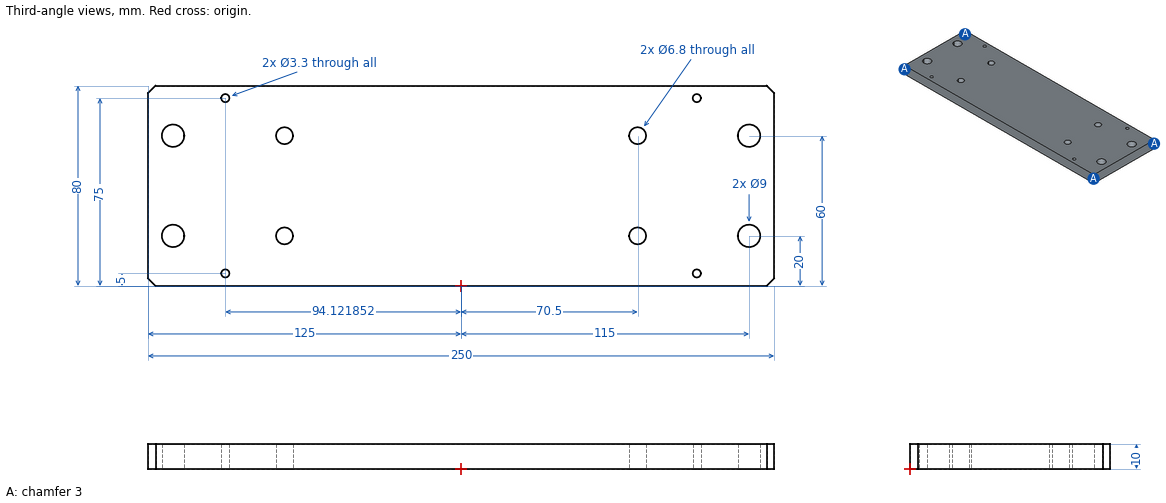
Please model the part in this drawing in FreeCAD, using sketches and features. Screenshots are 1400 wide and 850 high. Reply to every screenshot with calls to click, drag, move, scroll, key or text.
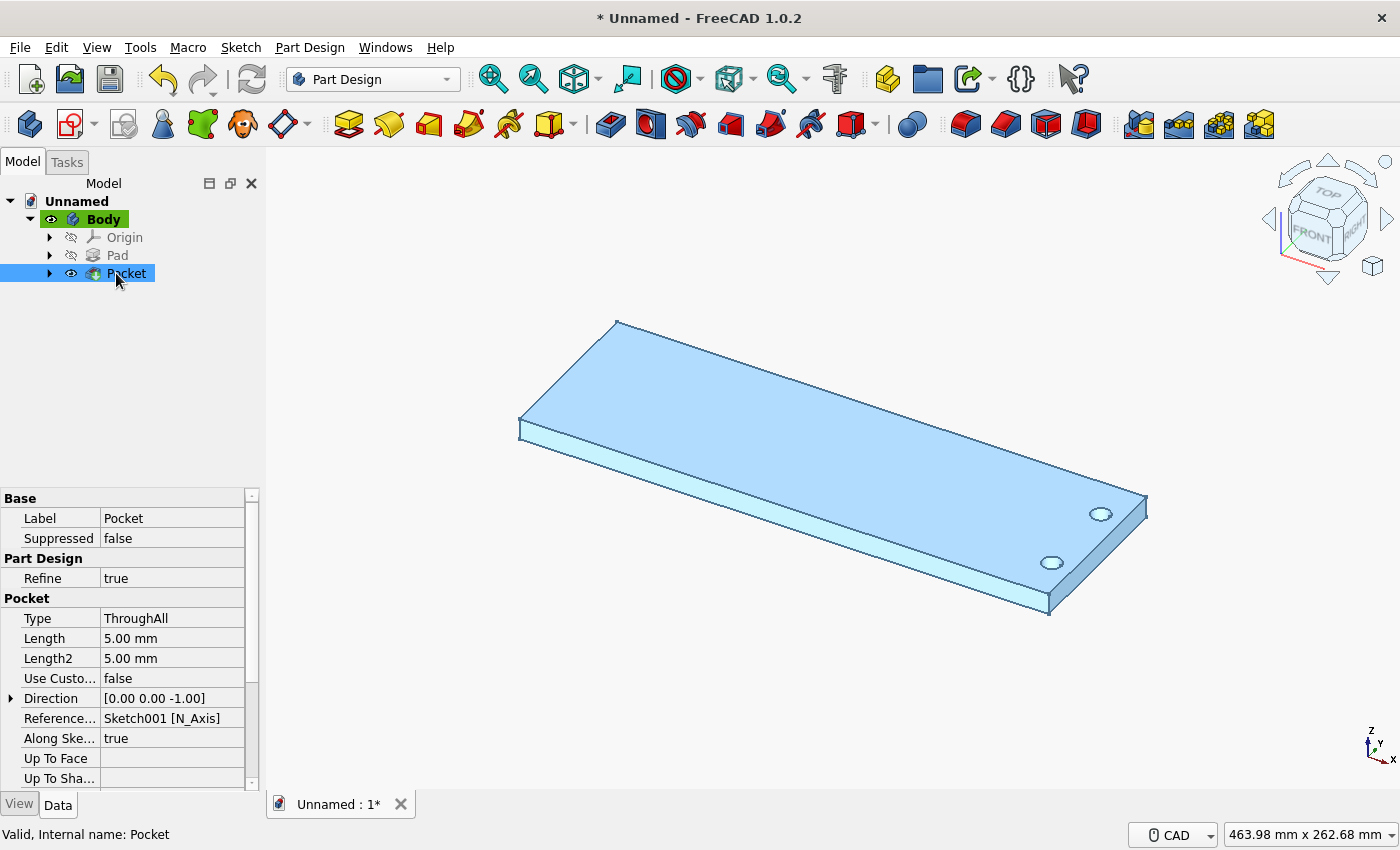
click(1140, 124)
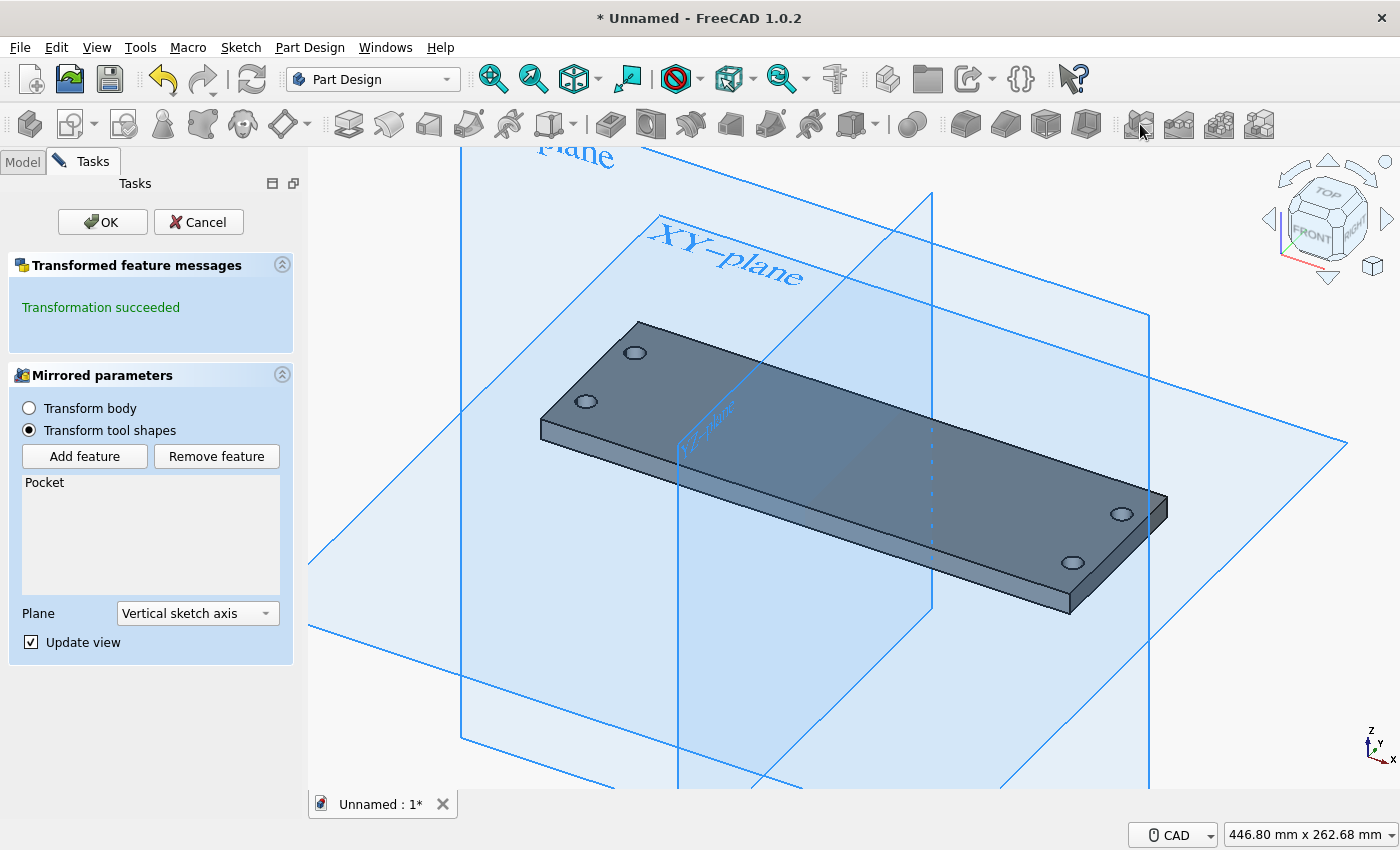
click(198, 614)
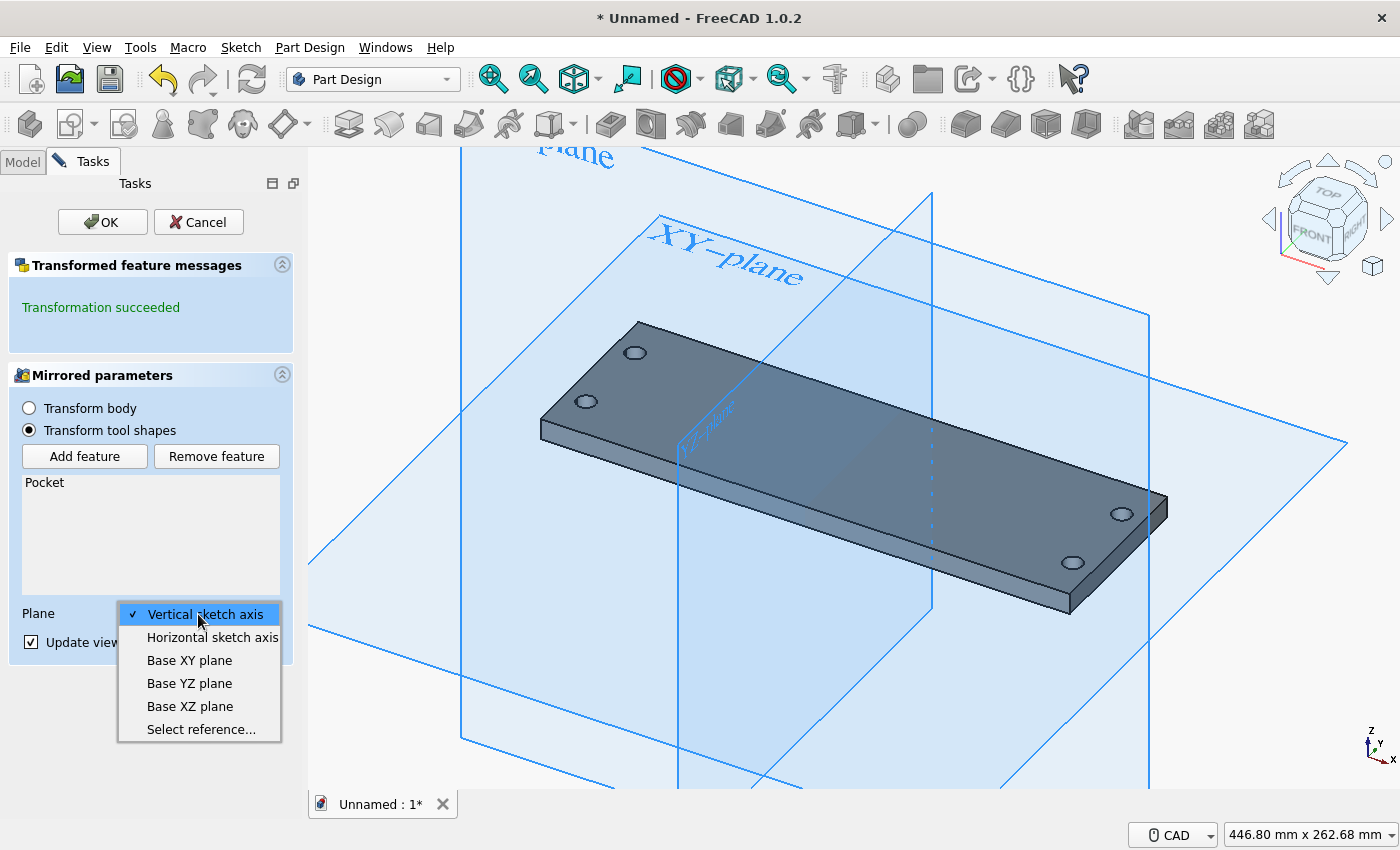
click(198, 684)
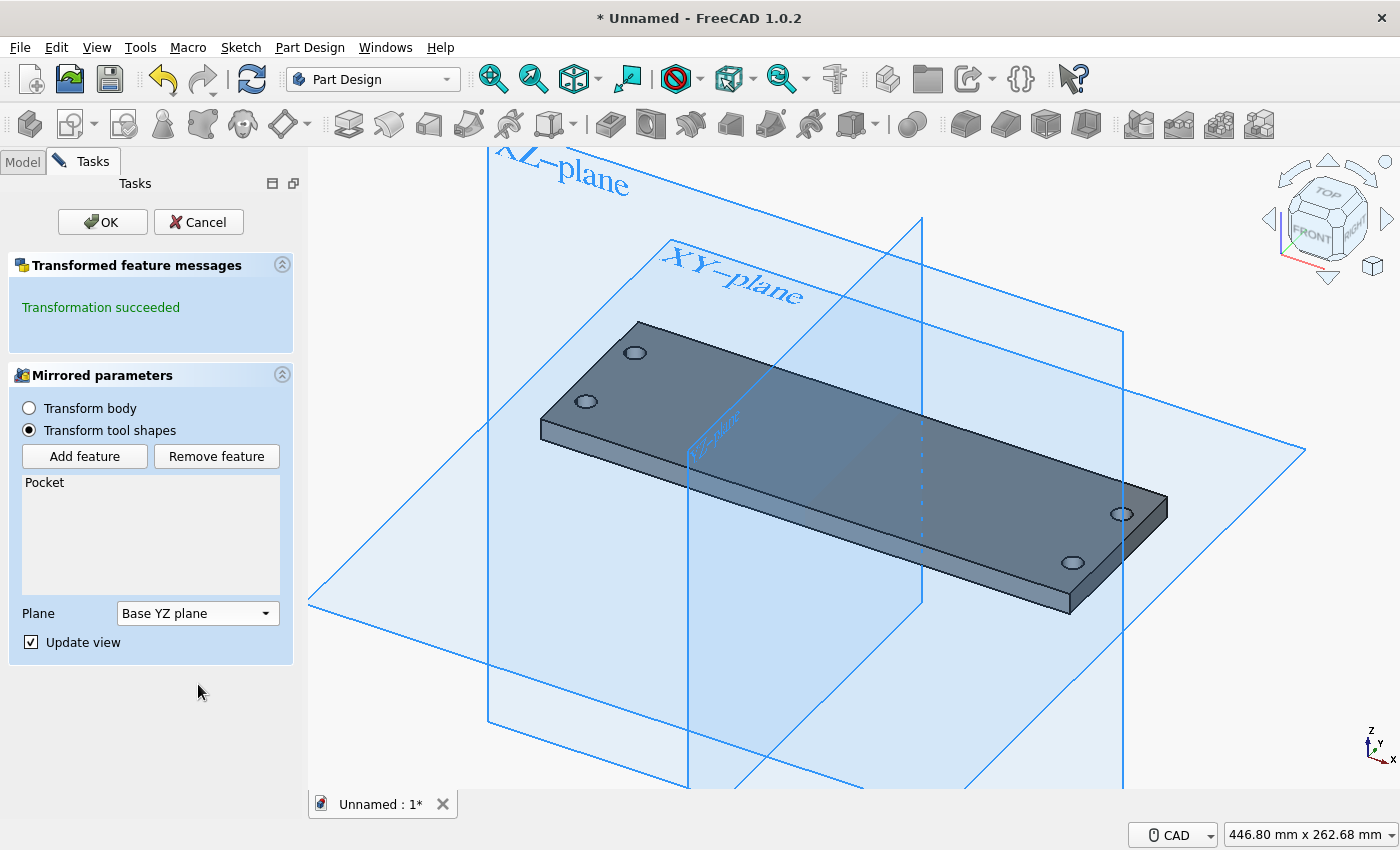
click(103, 222)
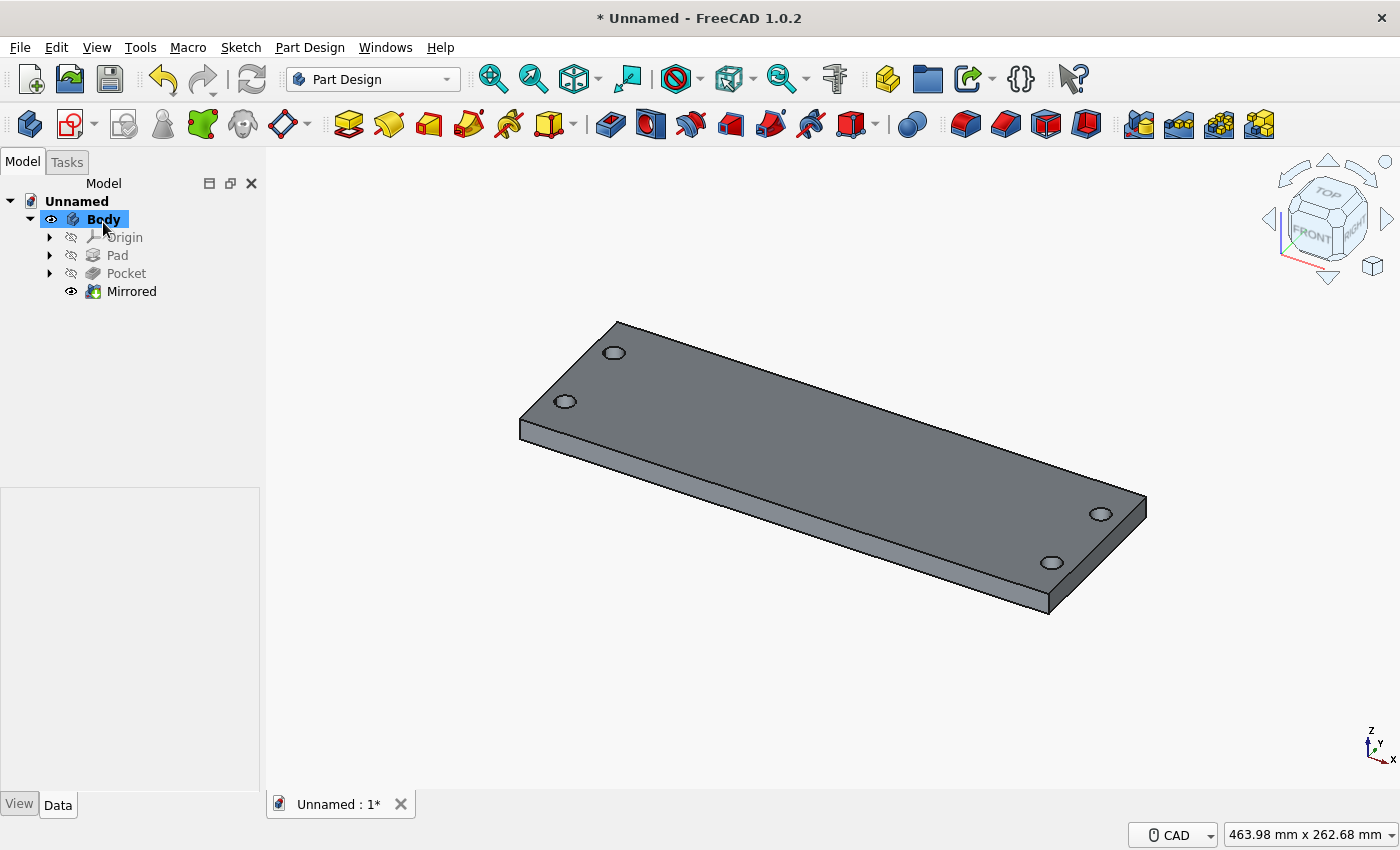
click(1049, 603)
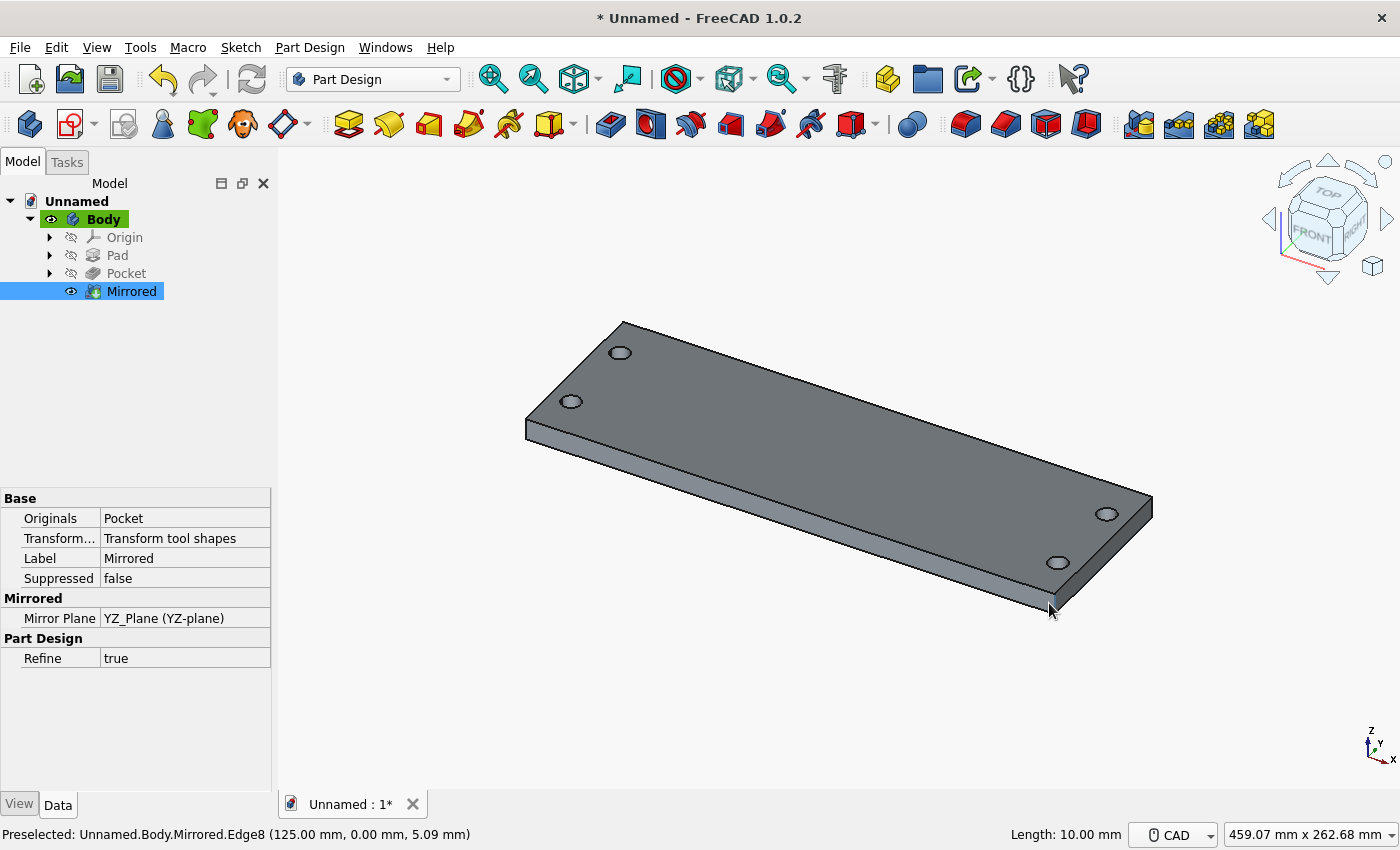
key(0)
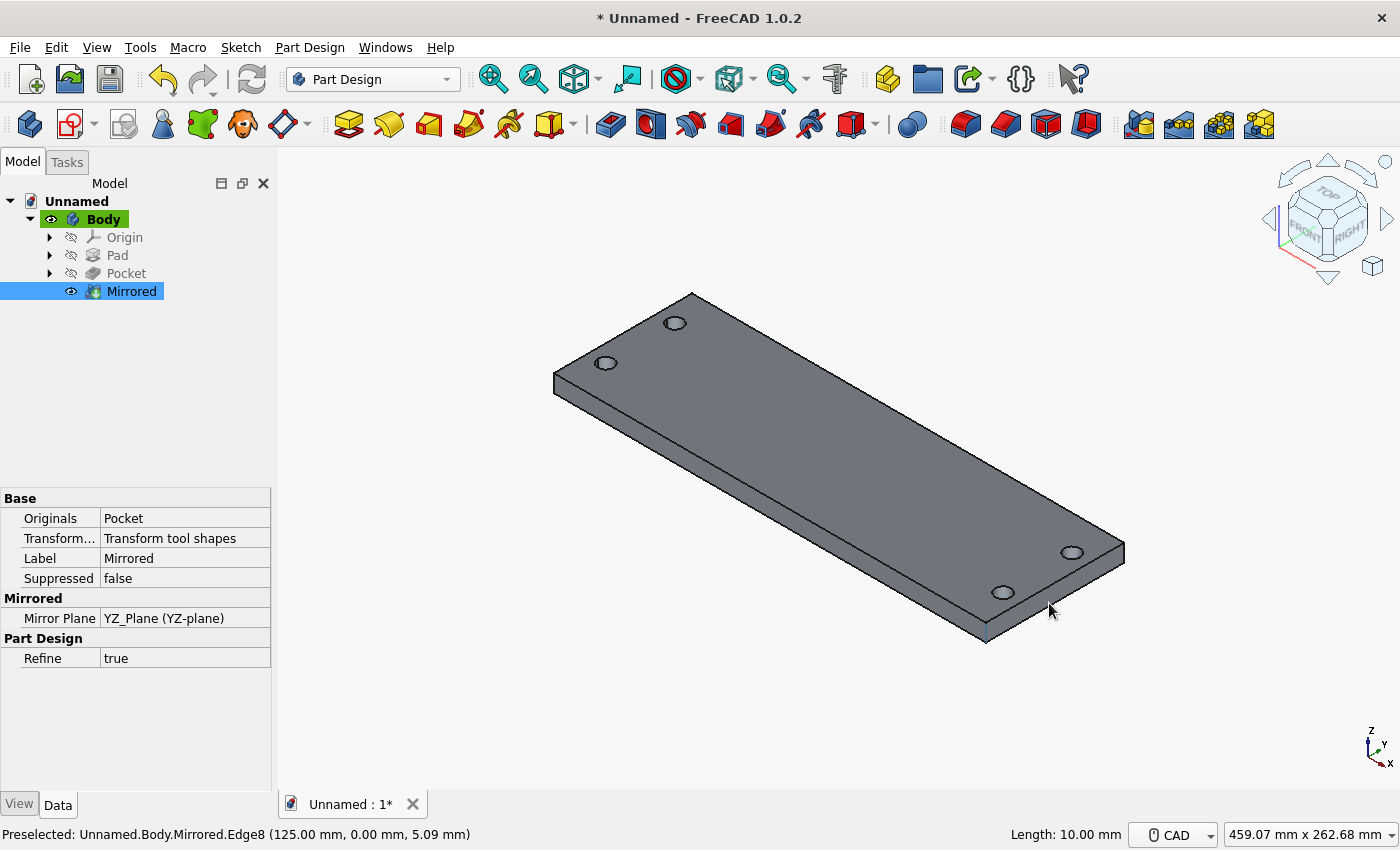
key(2)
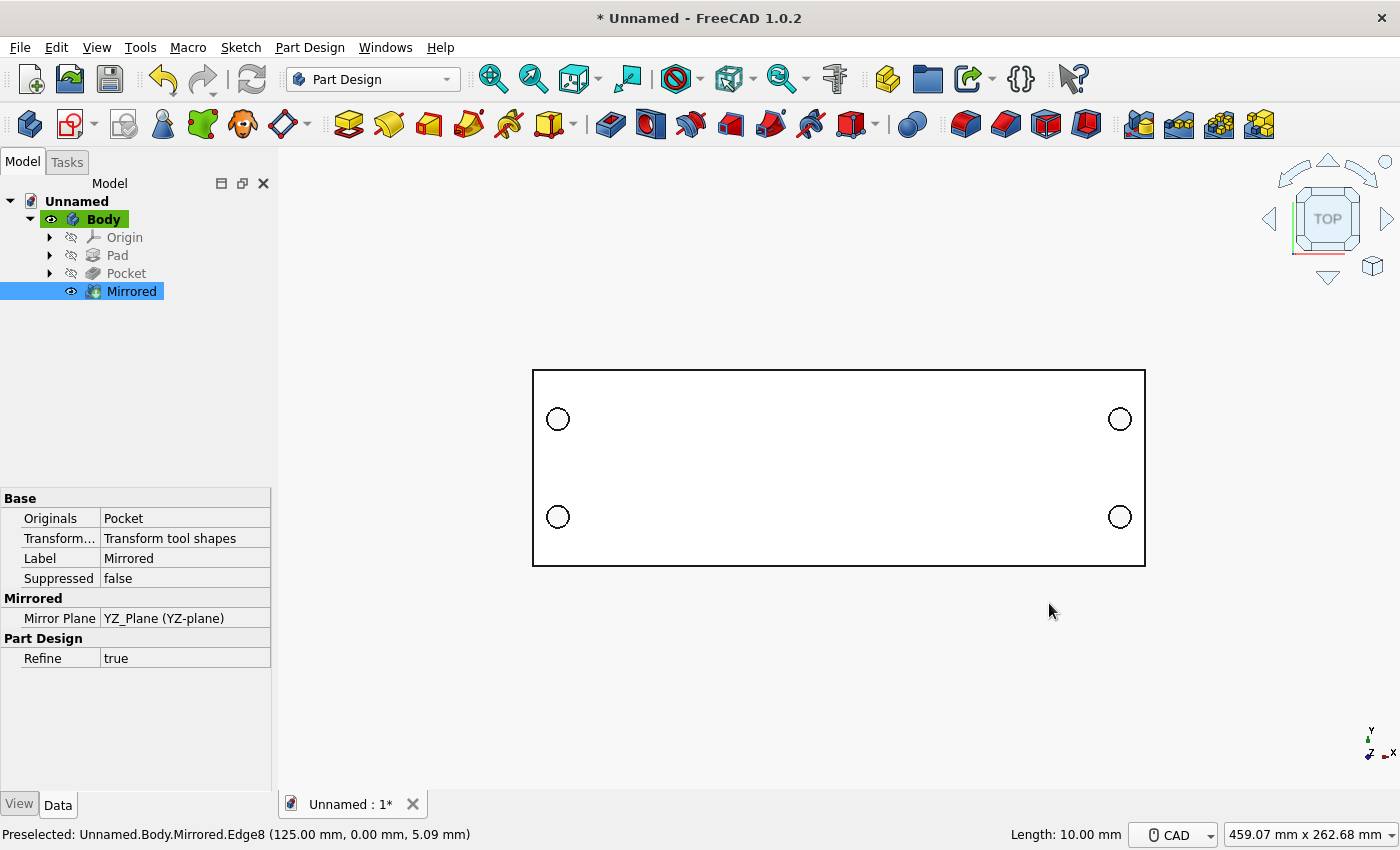
key(1)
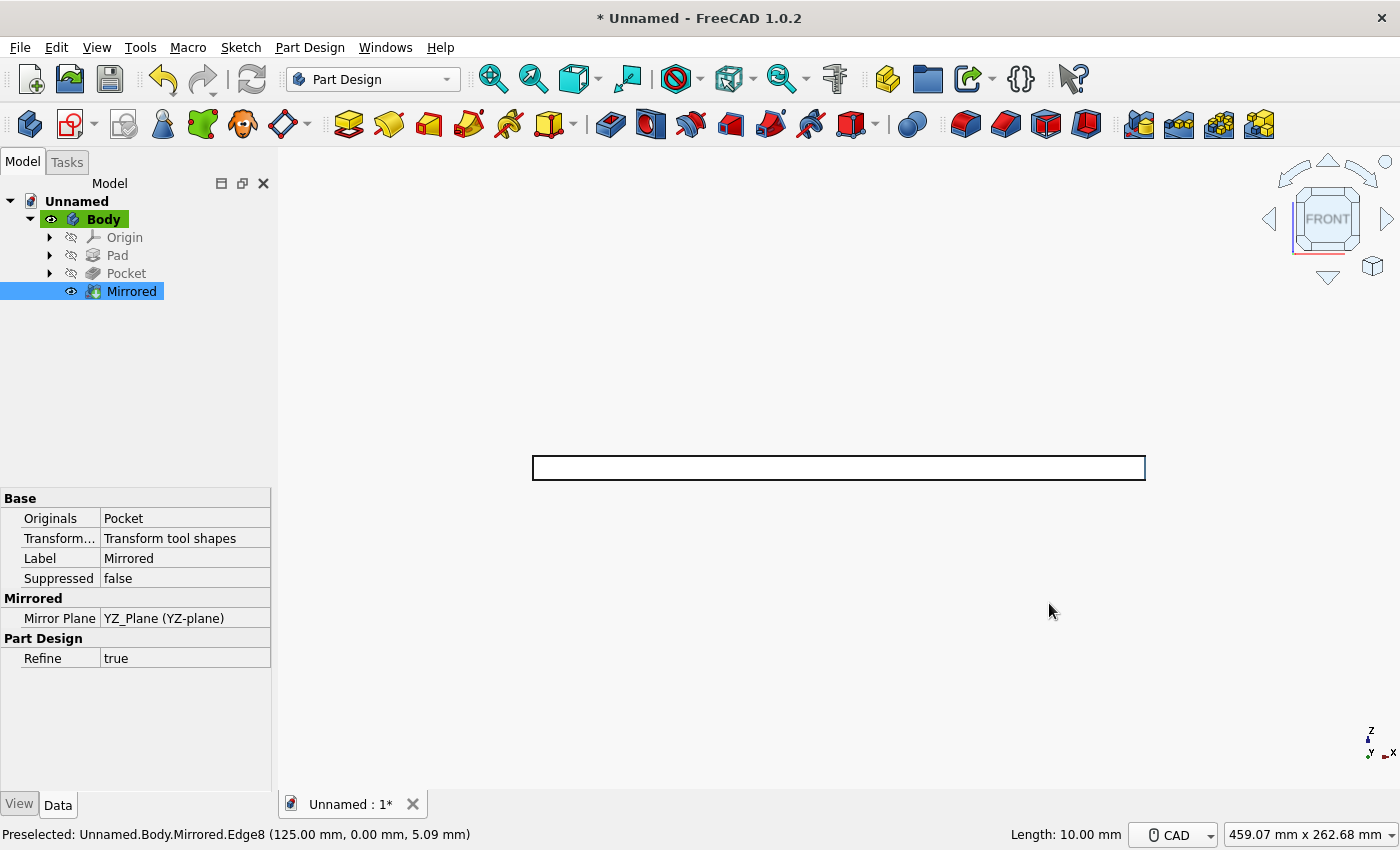
click(533, 467, ctrl)